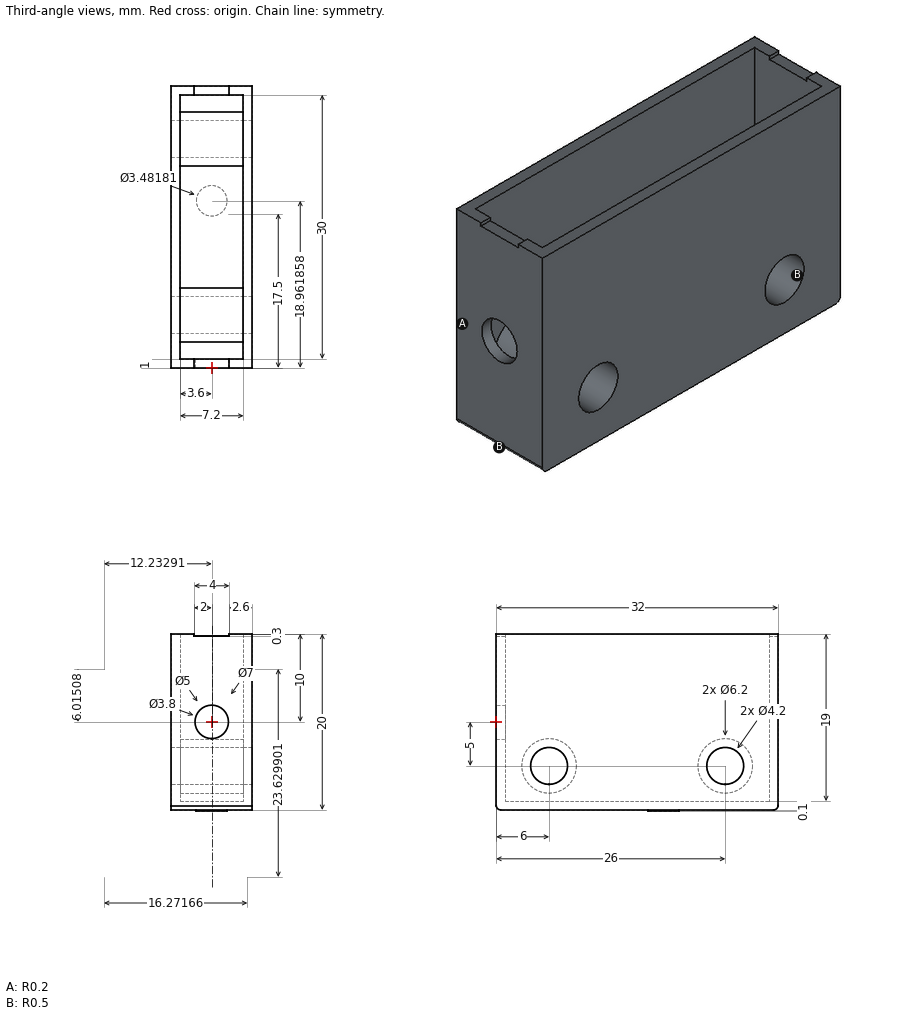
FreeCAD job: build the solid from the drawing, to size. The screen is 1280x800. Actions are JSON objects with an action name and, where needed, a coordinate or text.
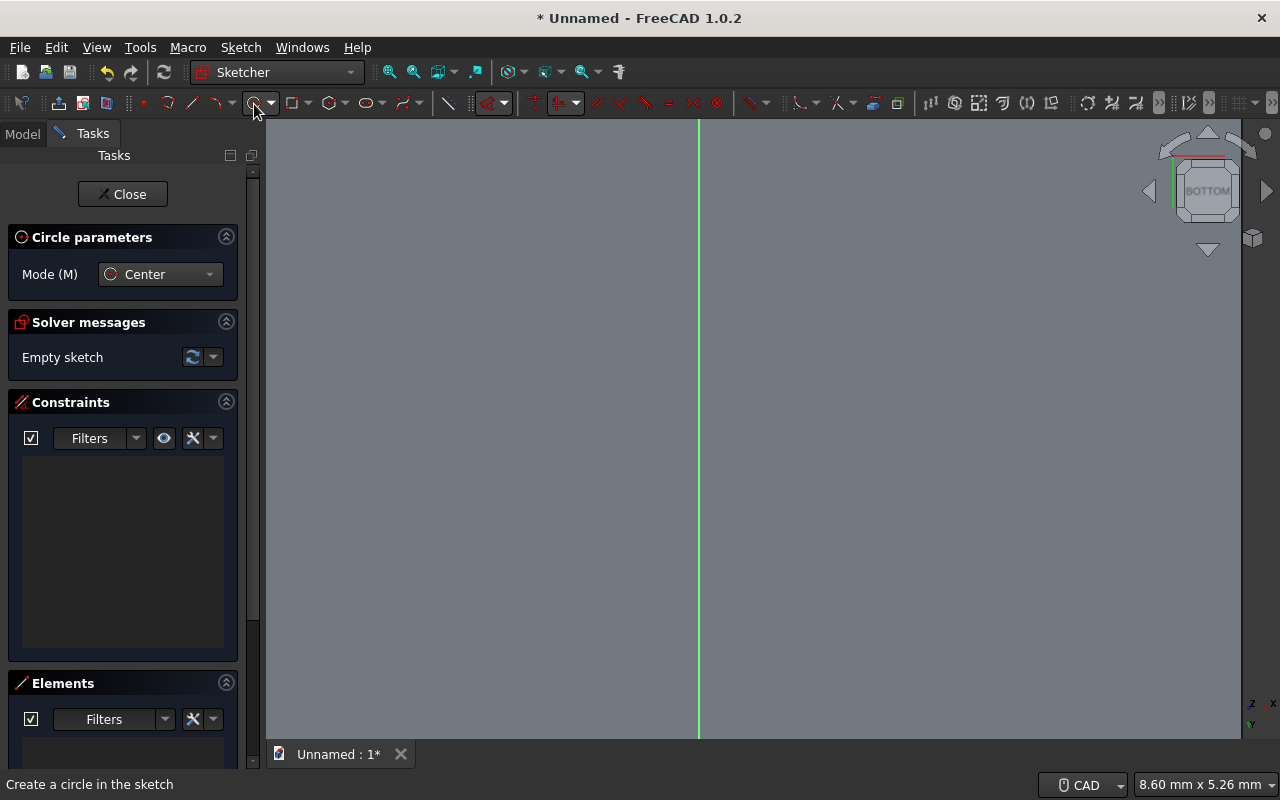
{"action": "left_click", "coordinate": [699, 423]}
{"action": "mouse_move", "coordinate": [845, 278]}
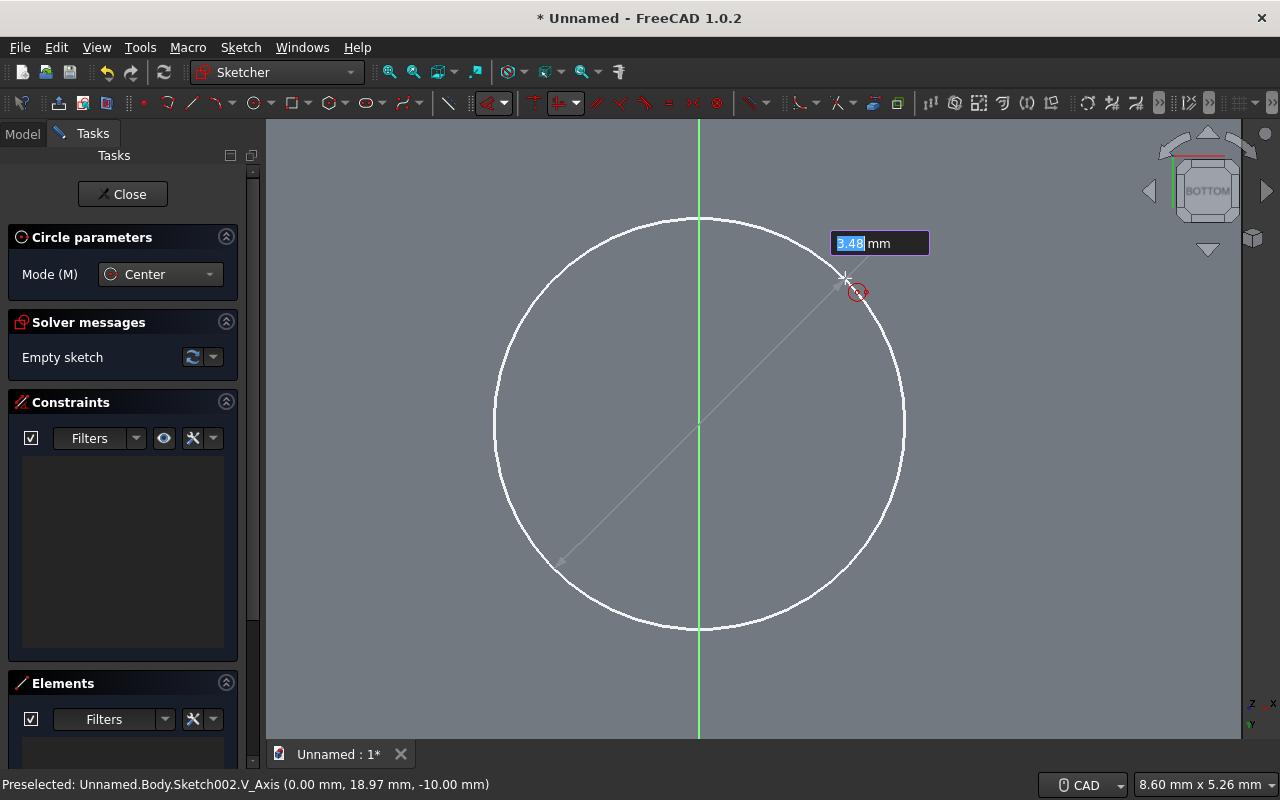
{"action": "type", "text": "3.48181"}
{"action": "key", "text": "Return"}
{"action": "key", "text": "Escape"}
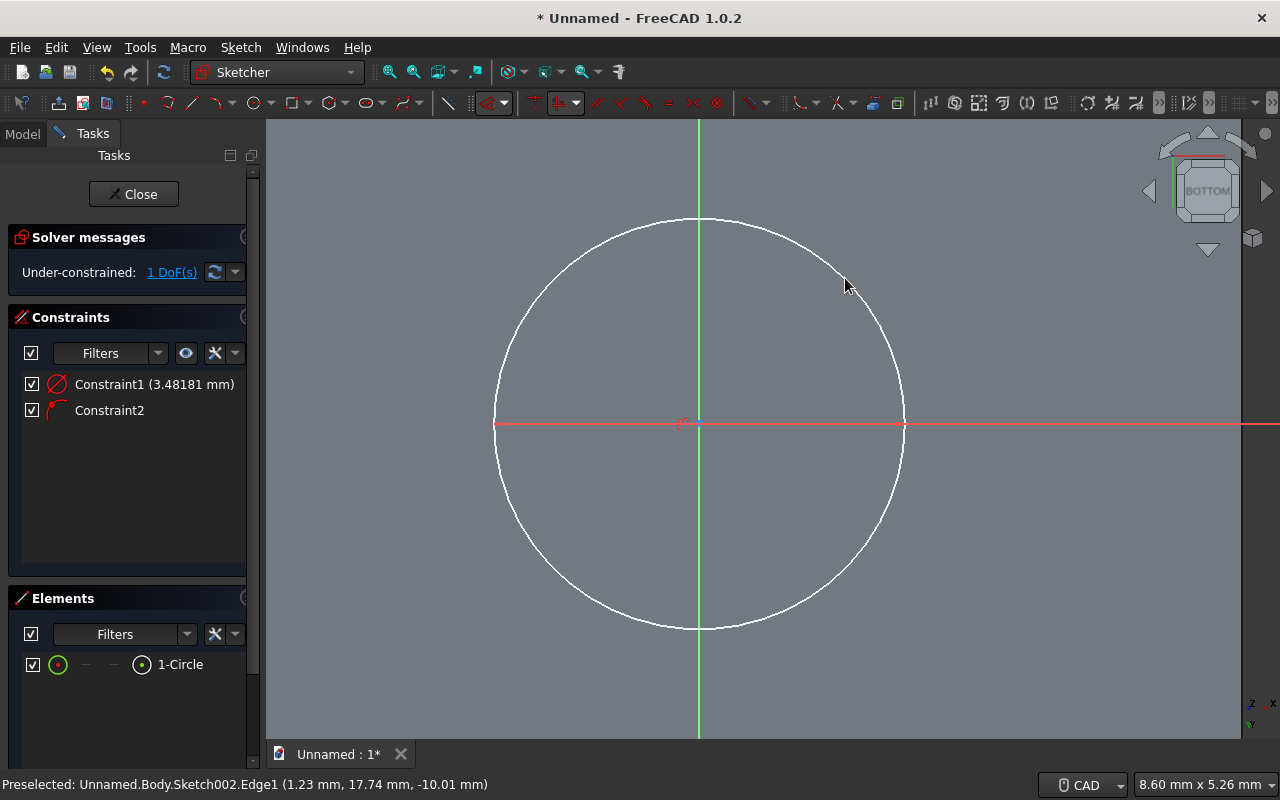
{"action": "left_click", "coordinate": [699, 424]}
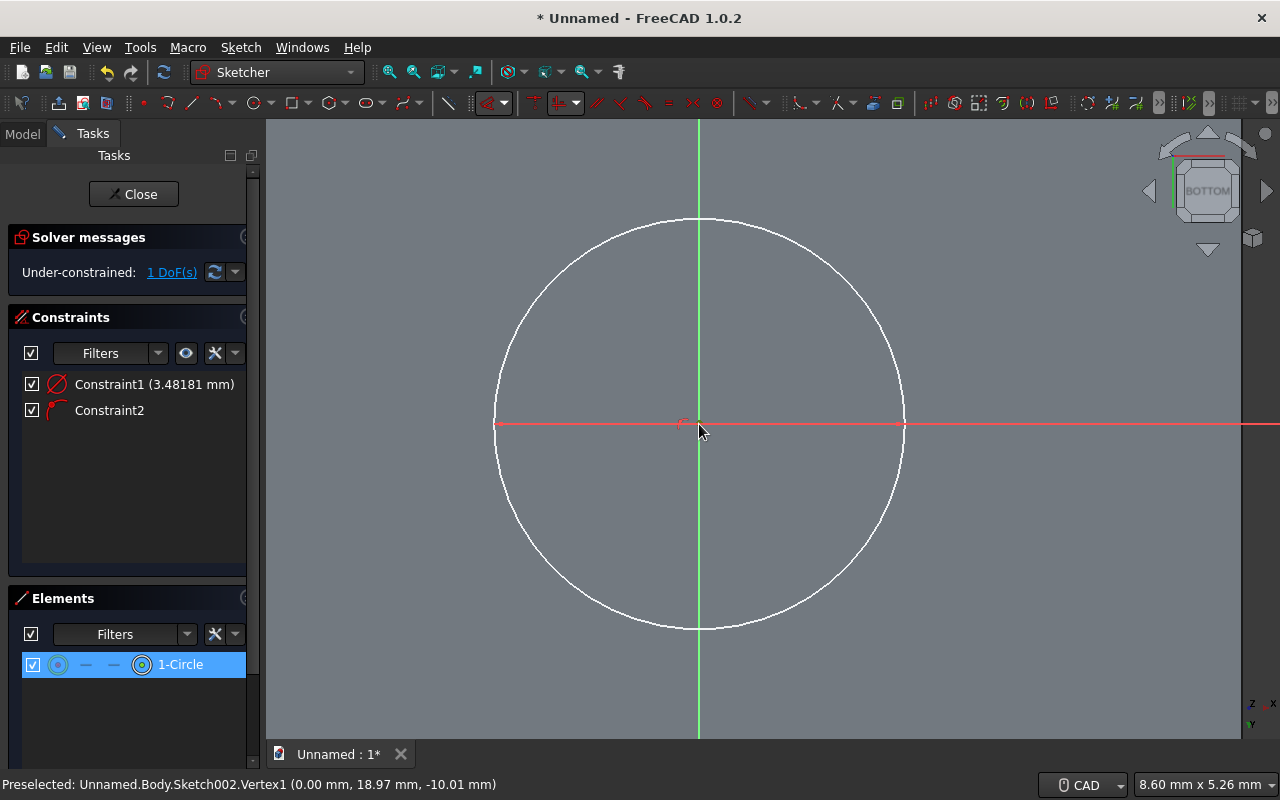
{"action": "key", "text": "i"}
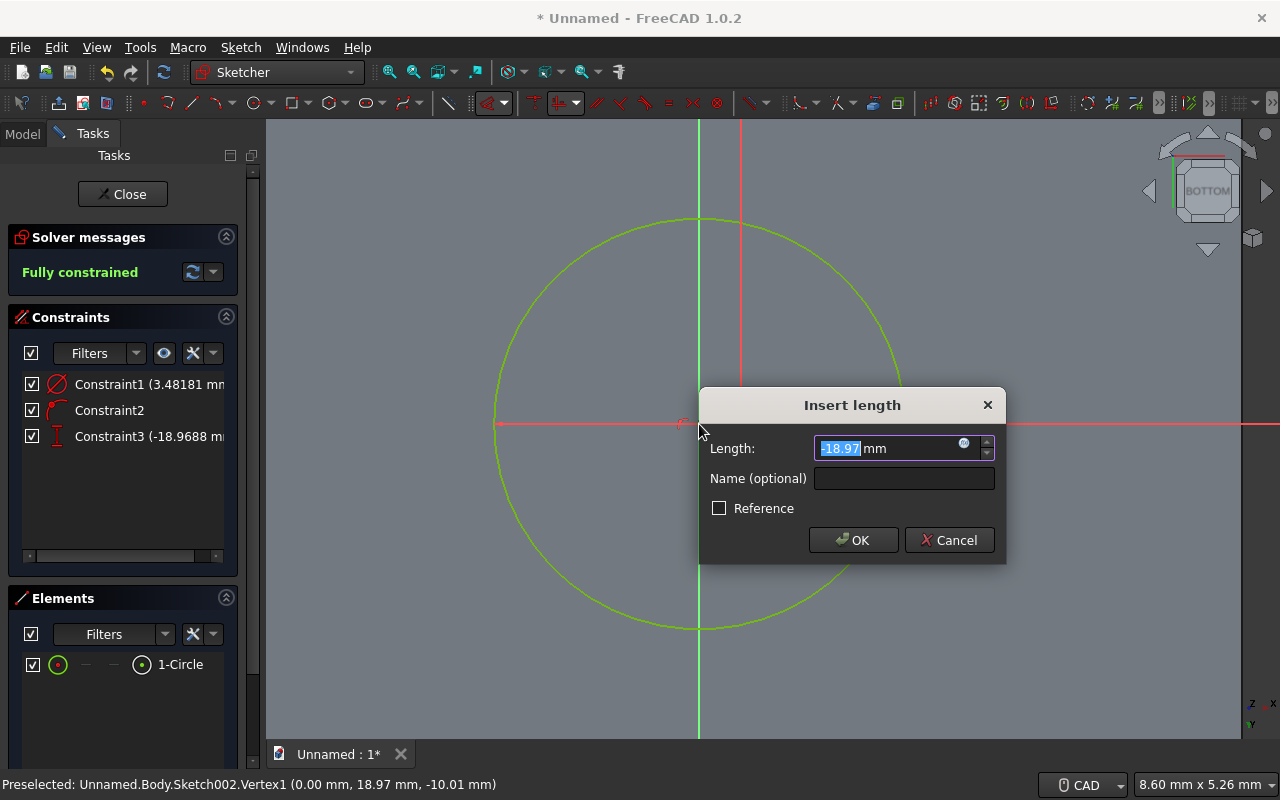
{"action": "type", "text": "-18.961858"}
{"action": "key", "text": "Return"}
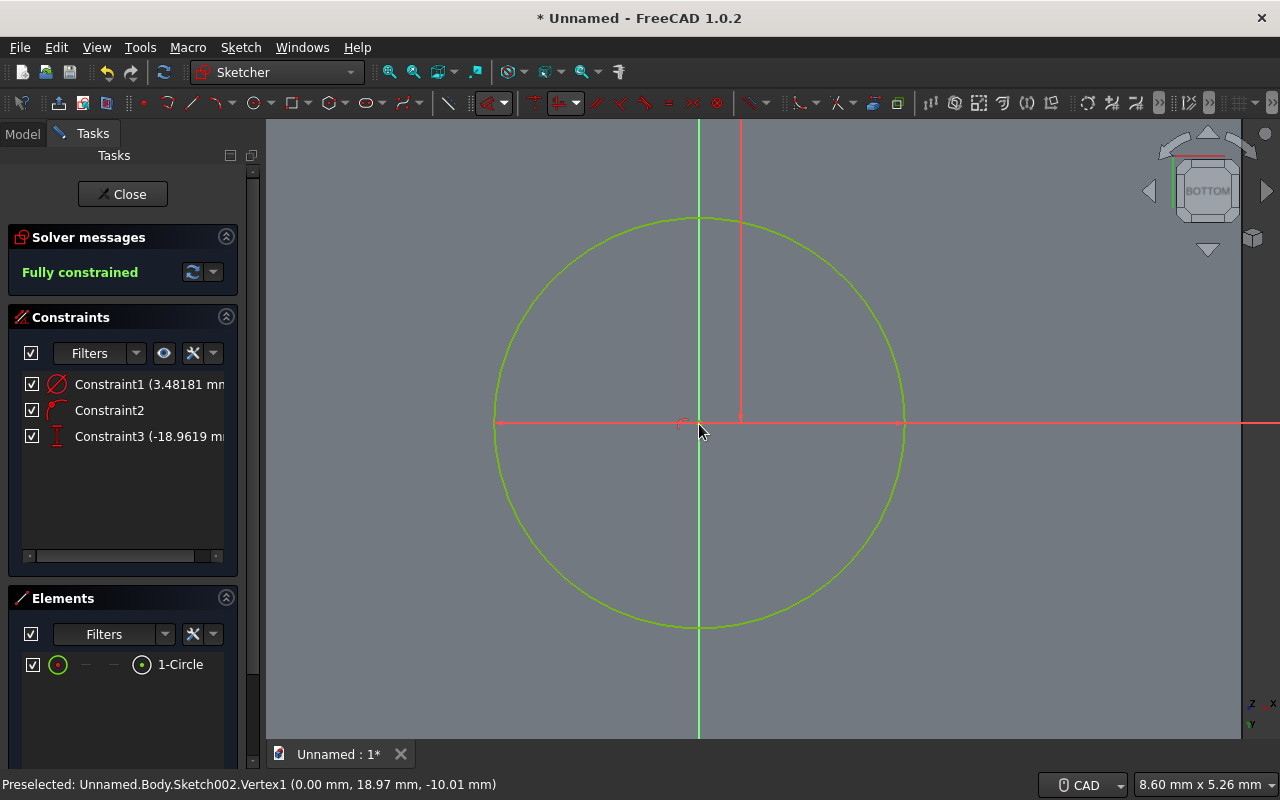
{"action": "left_click", "coordinate": [123, 194]}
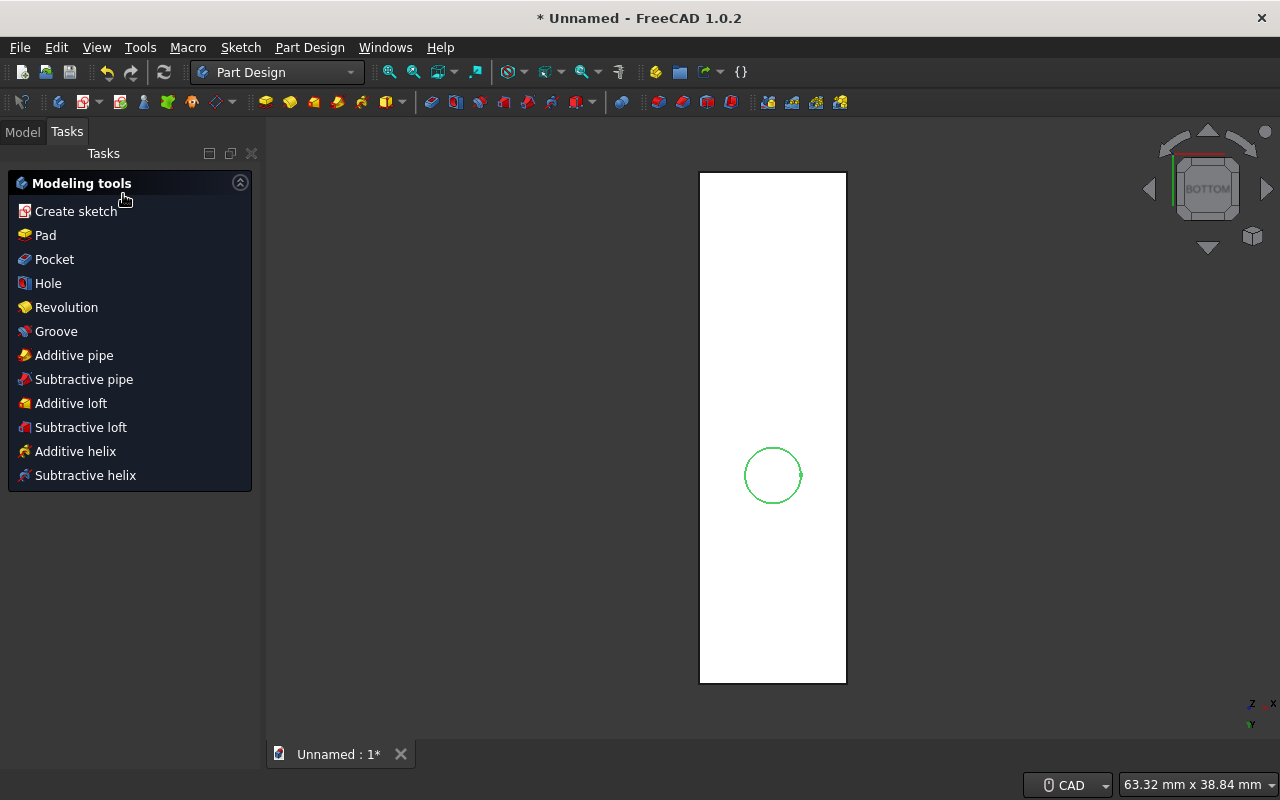
{"action": "left_click", "coordinate": [266, 102]}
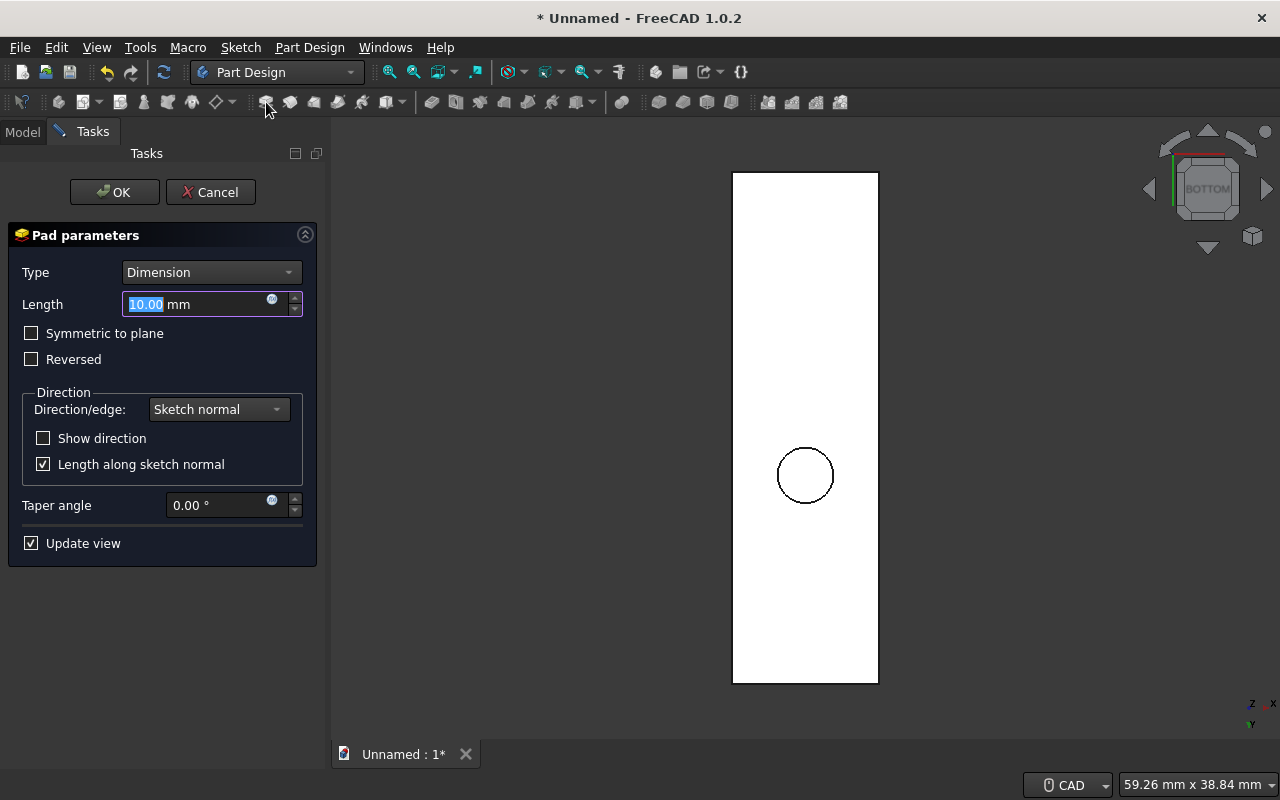
{"action": "type", "text": "0.1"}
{"action": "key", "text": "Tab"}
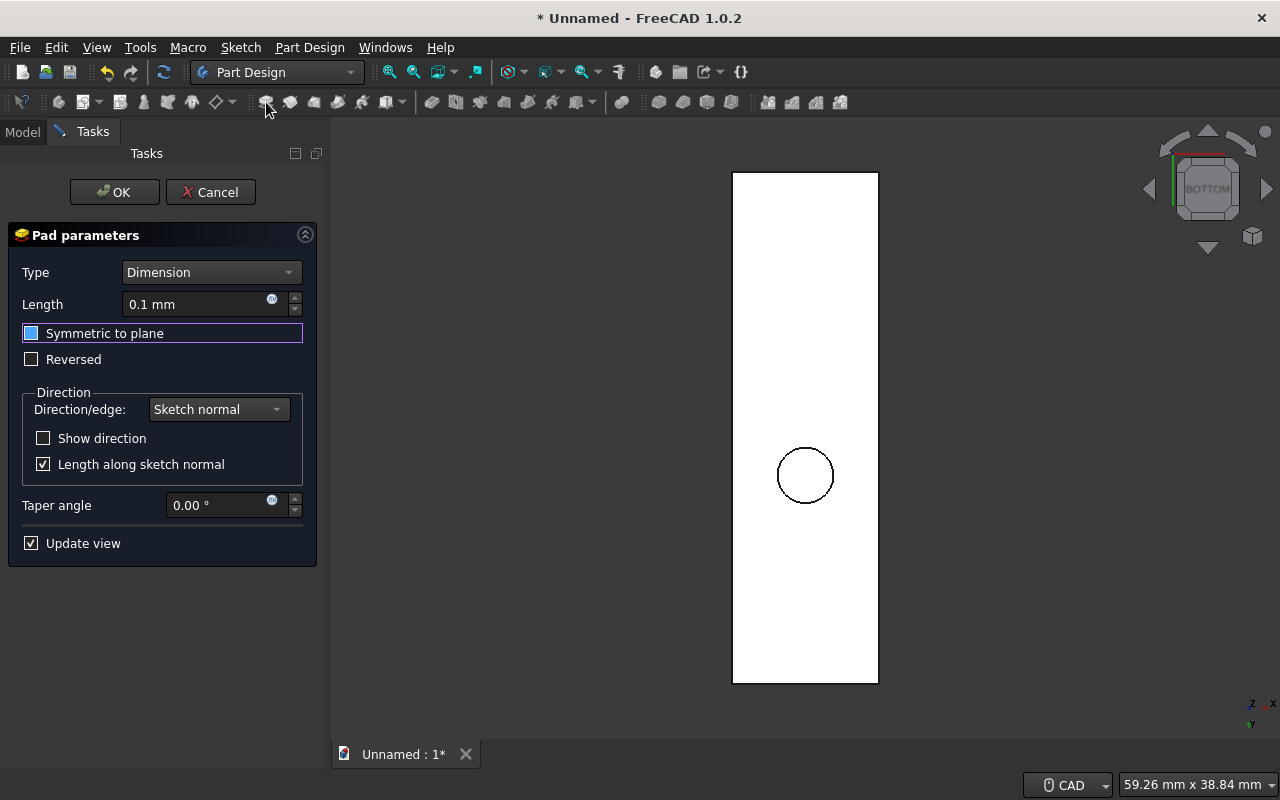
{"action": "left_click", "coordinate": [115, 192]}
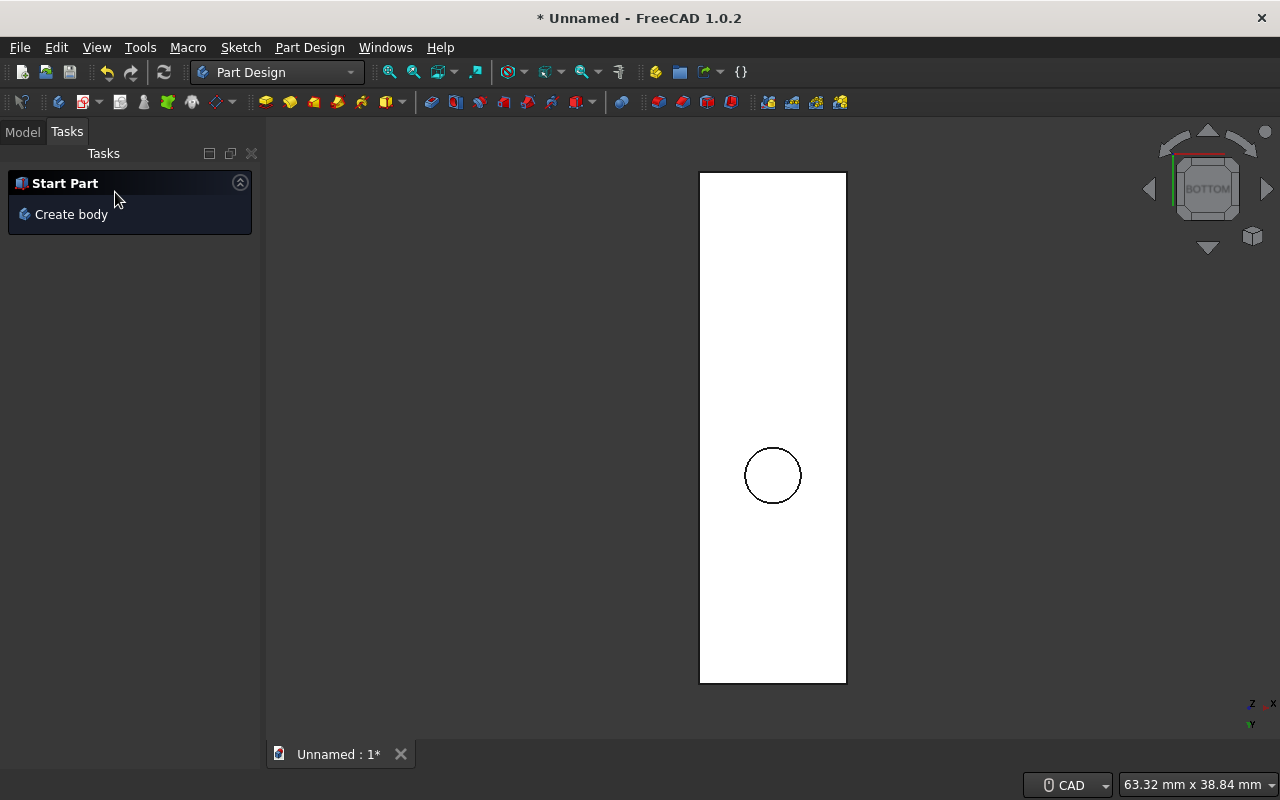
{"action": "key", "text": "0"}